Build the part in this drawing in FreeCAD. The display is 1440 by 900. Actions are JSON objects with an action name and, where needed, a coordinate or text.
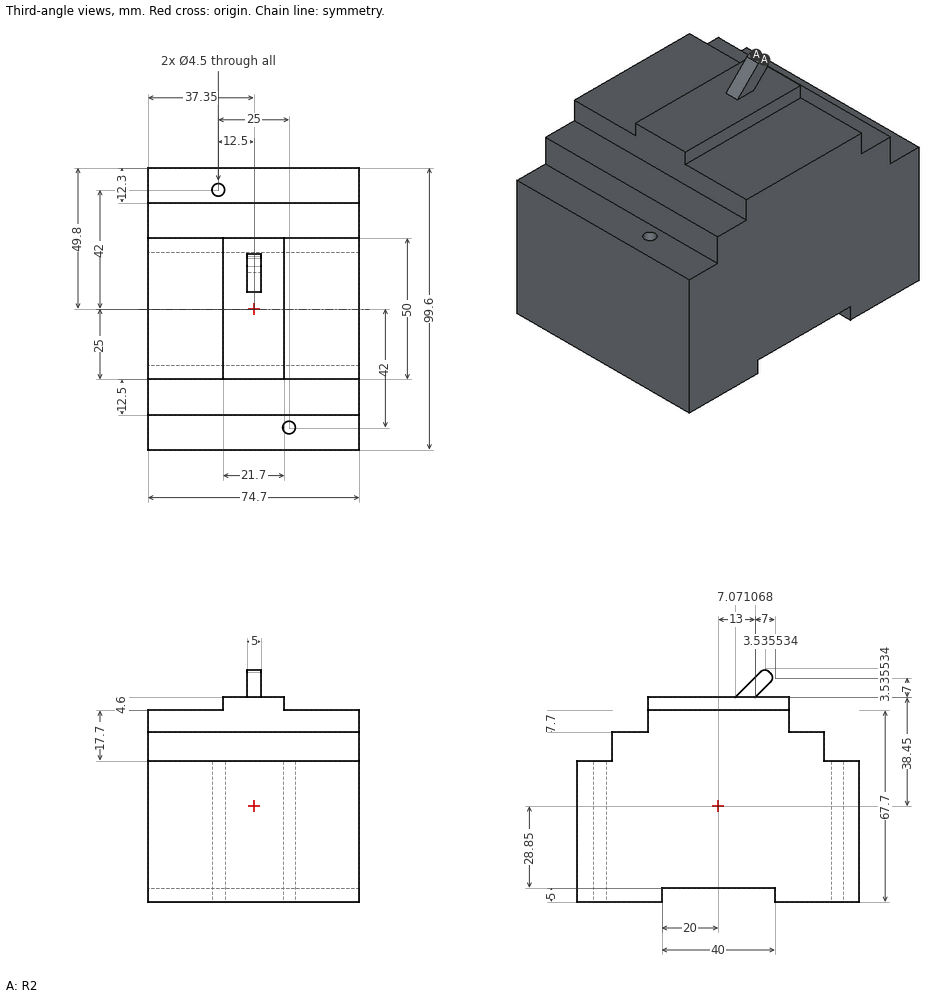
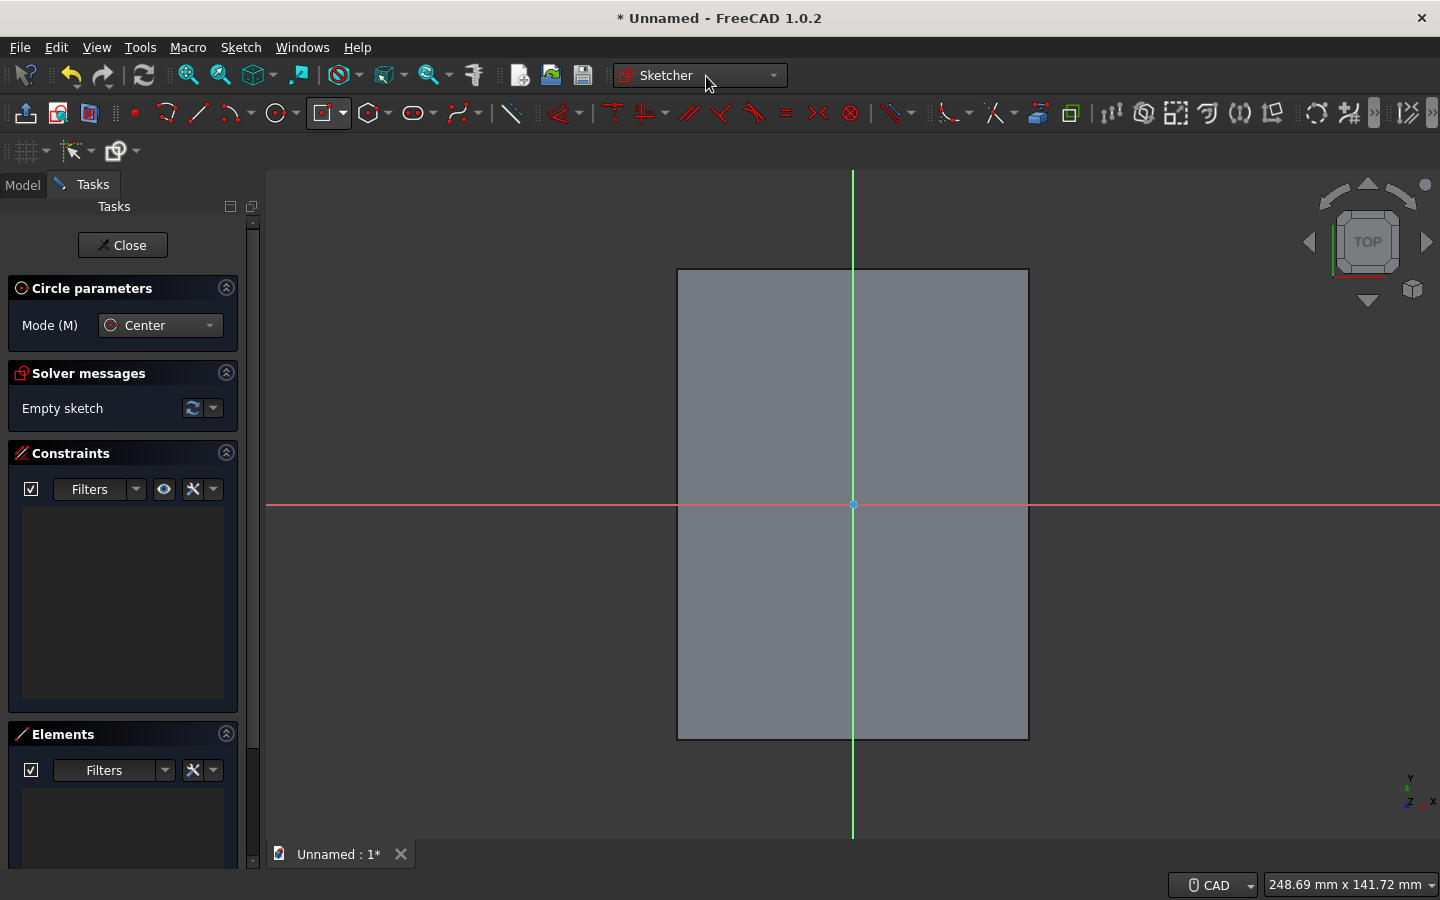
{"action": "scroll", "coordinate": [794, 306], "scroll_direction": "up", "scroll_amount": 4}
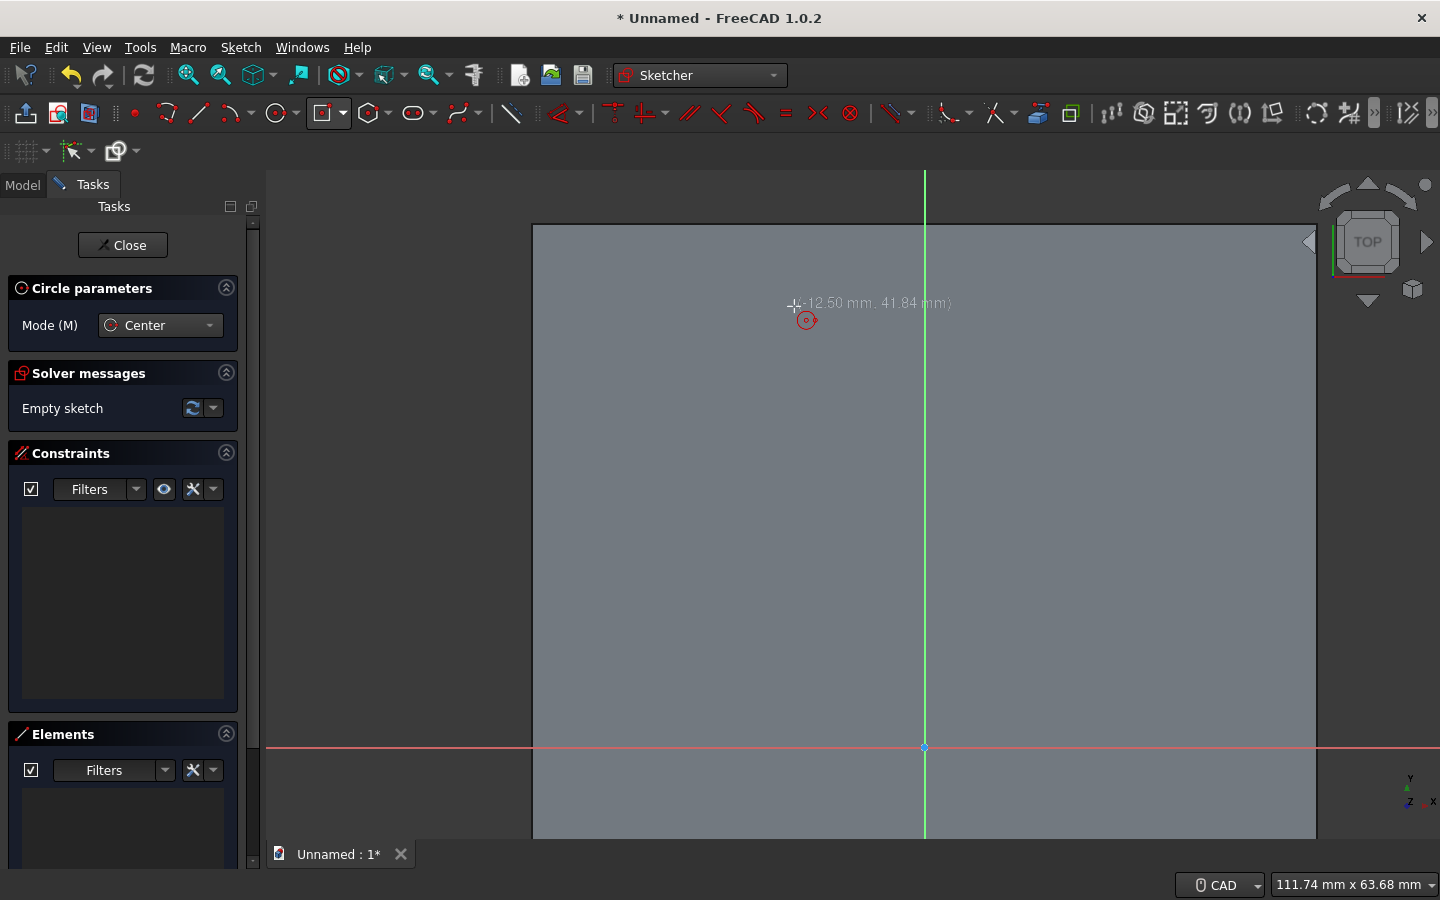
{"action": "left_click", "coordinate": [793, 306]}
{"action": "left_click", "coordinate": [810, 290]}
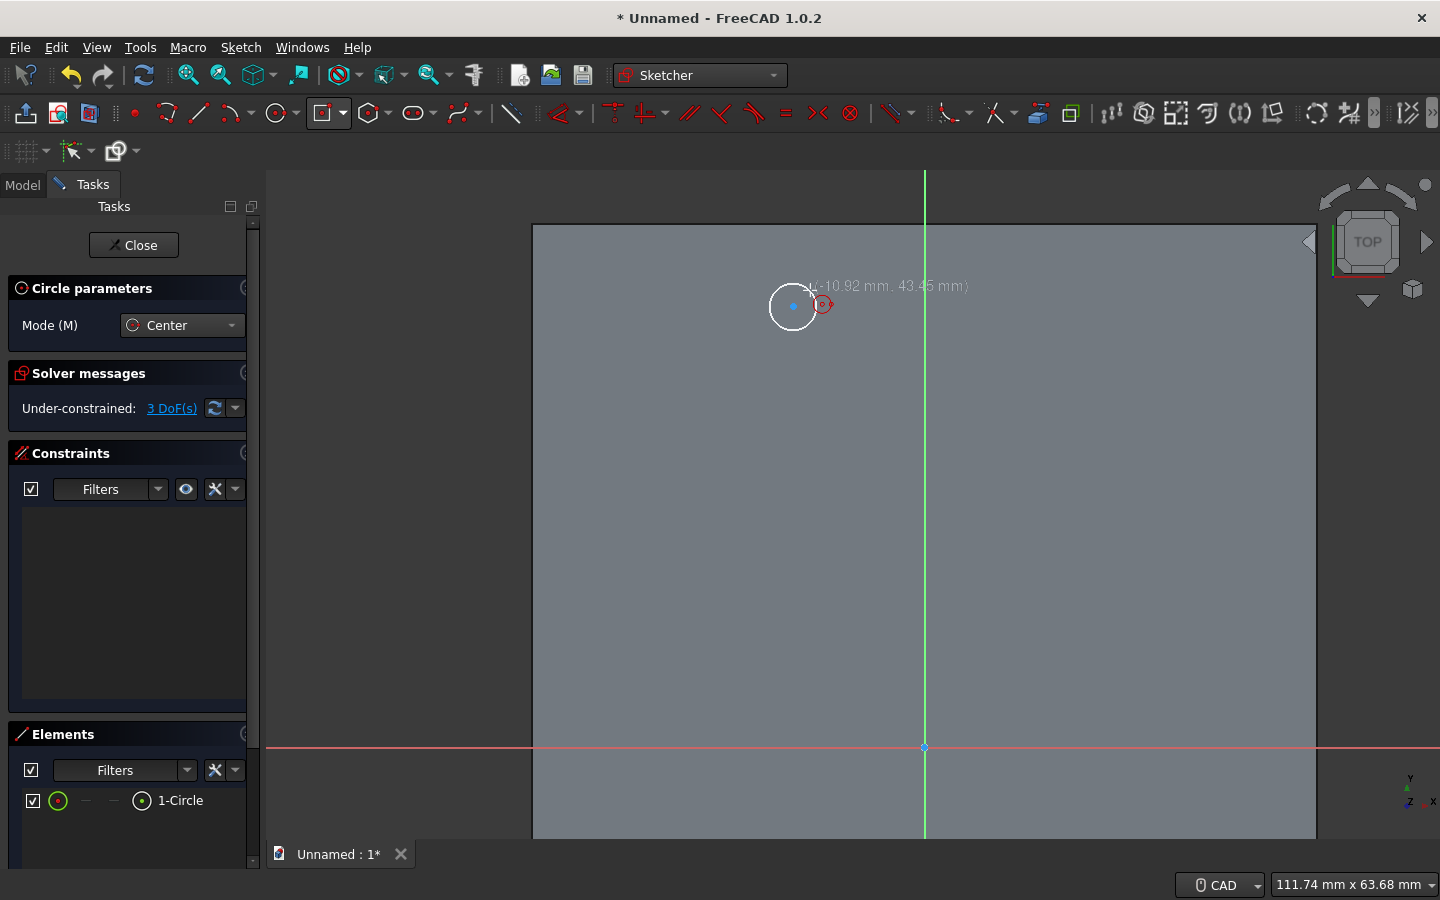
{"action": "scroll", "coordinate": [670, 306], "scroll_direction": "down", "scroll_amount": 4}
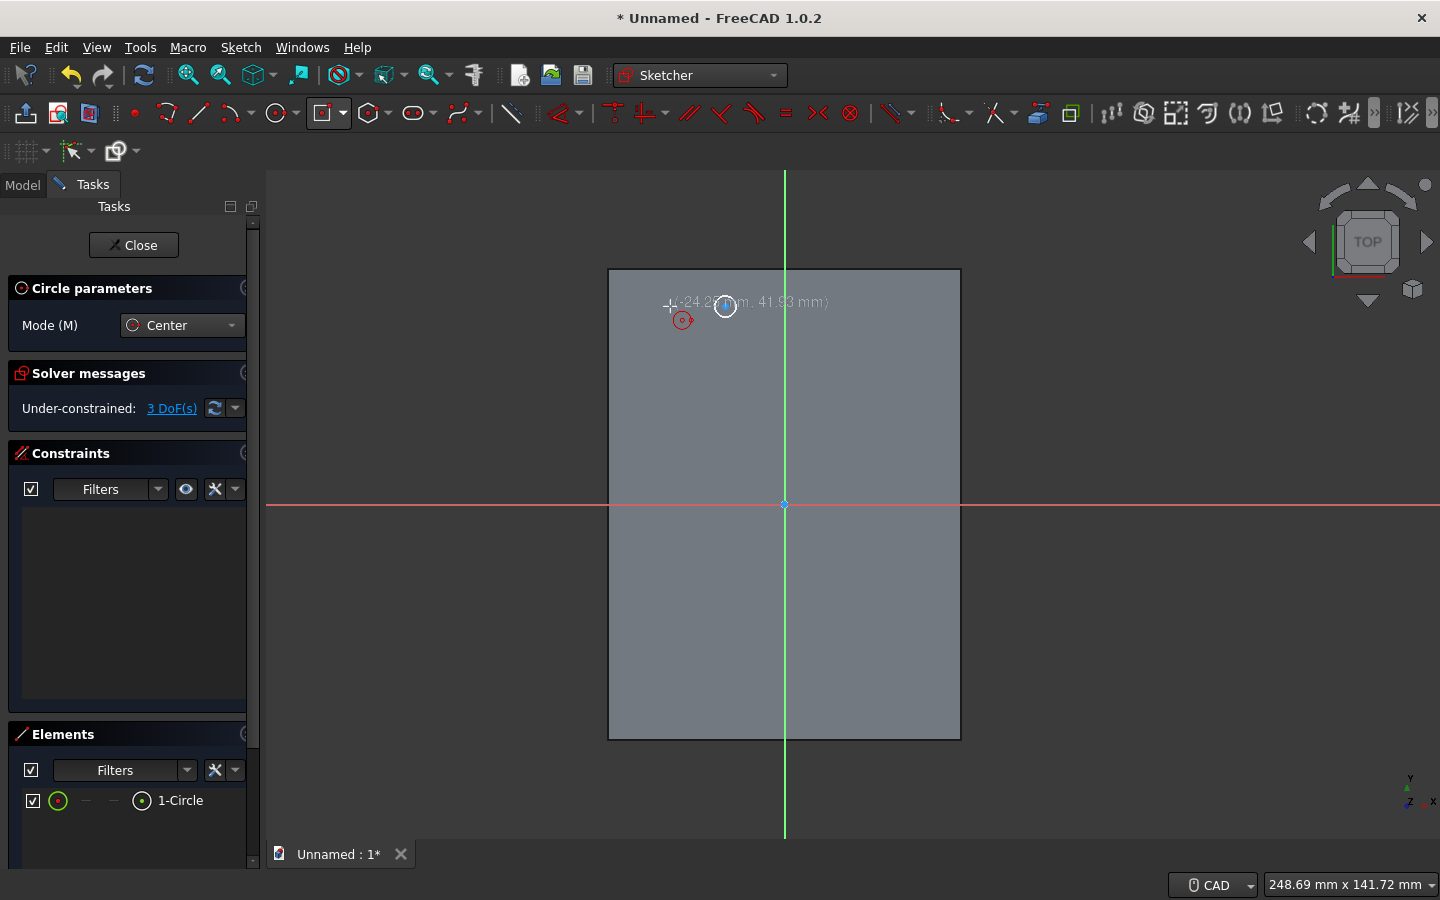
{"action": "scroll", "coordinate": [844, 703], "scroll_direction": "up", "scroll_amount": 4}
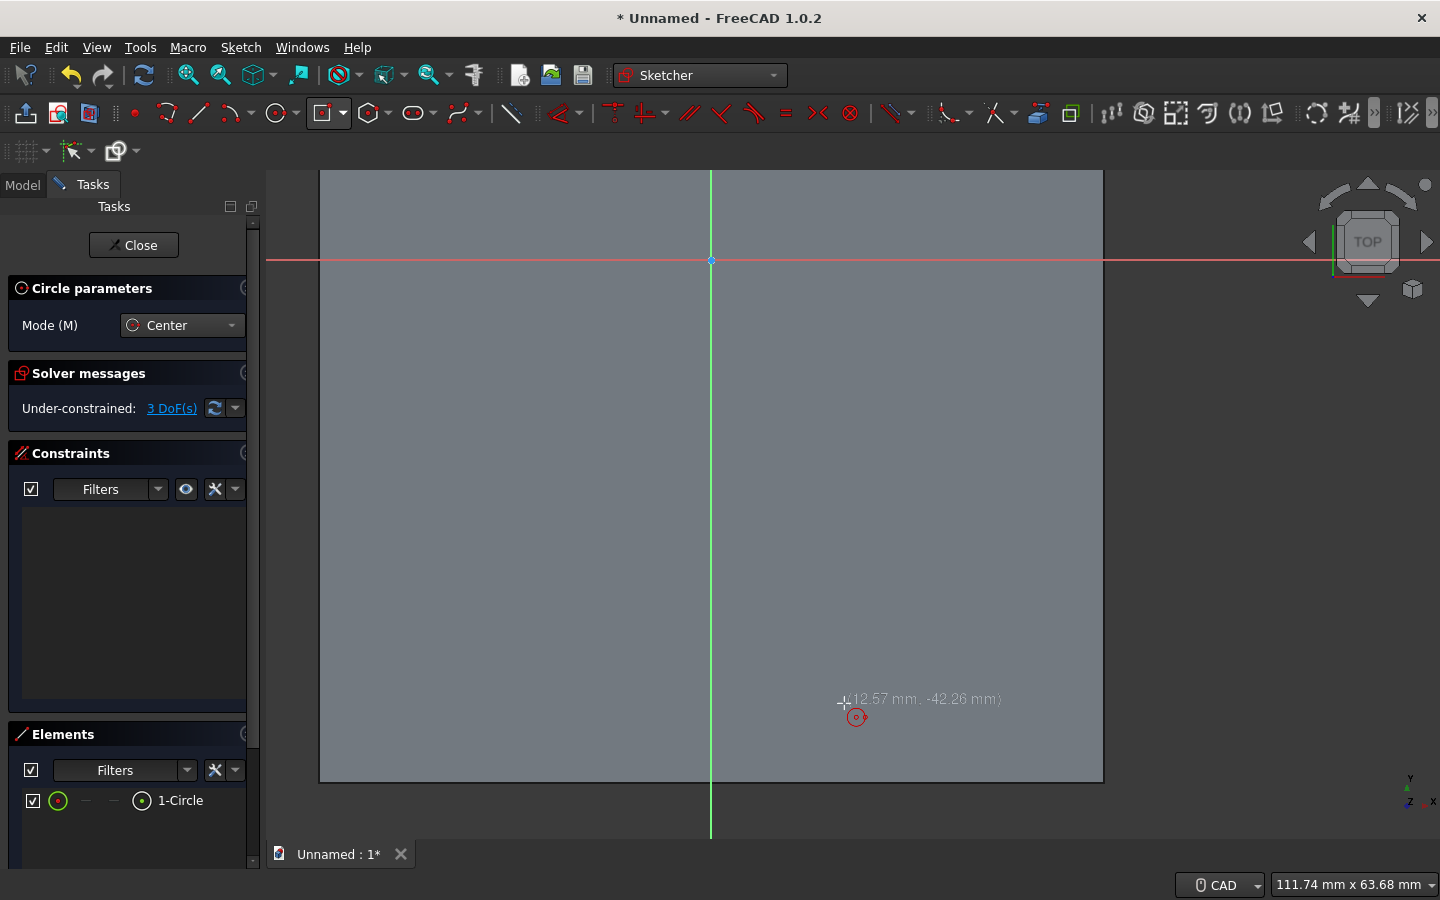
{"action": "left_click", "coordinate": [843, 702]}
{"action": "left_click", "coordinate": [859, 685]}
{"action": "key", "text": "Escape"}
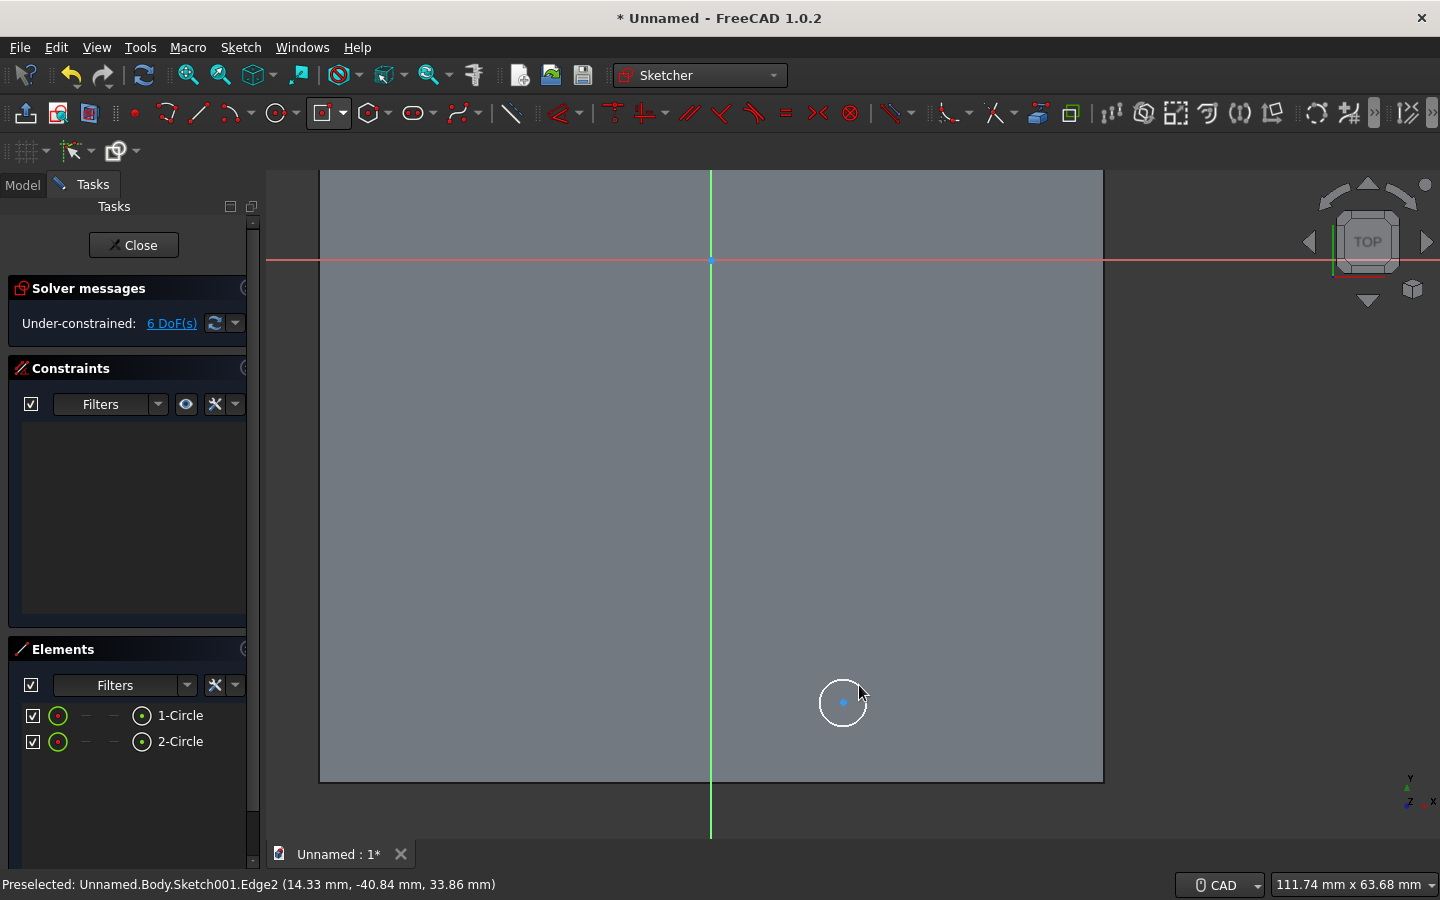
{"action": "scroll", "coordinate": [844, 704], "scroll_direction": "down", "scroll_amount": 4}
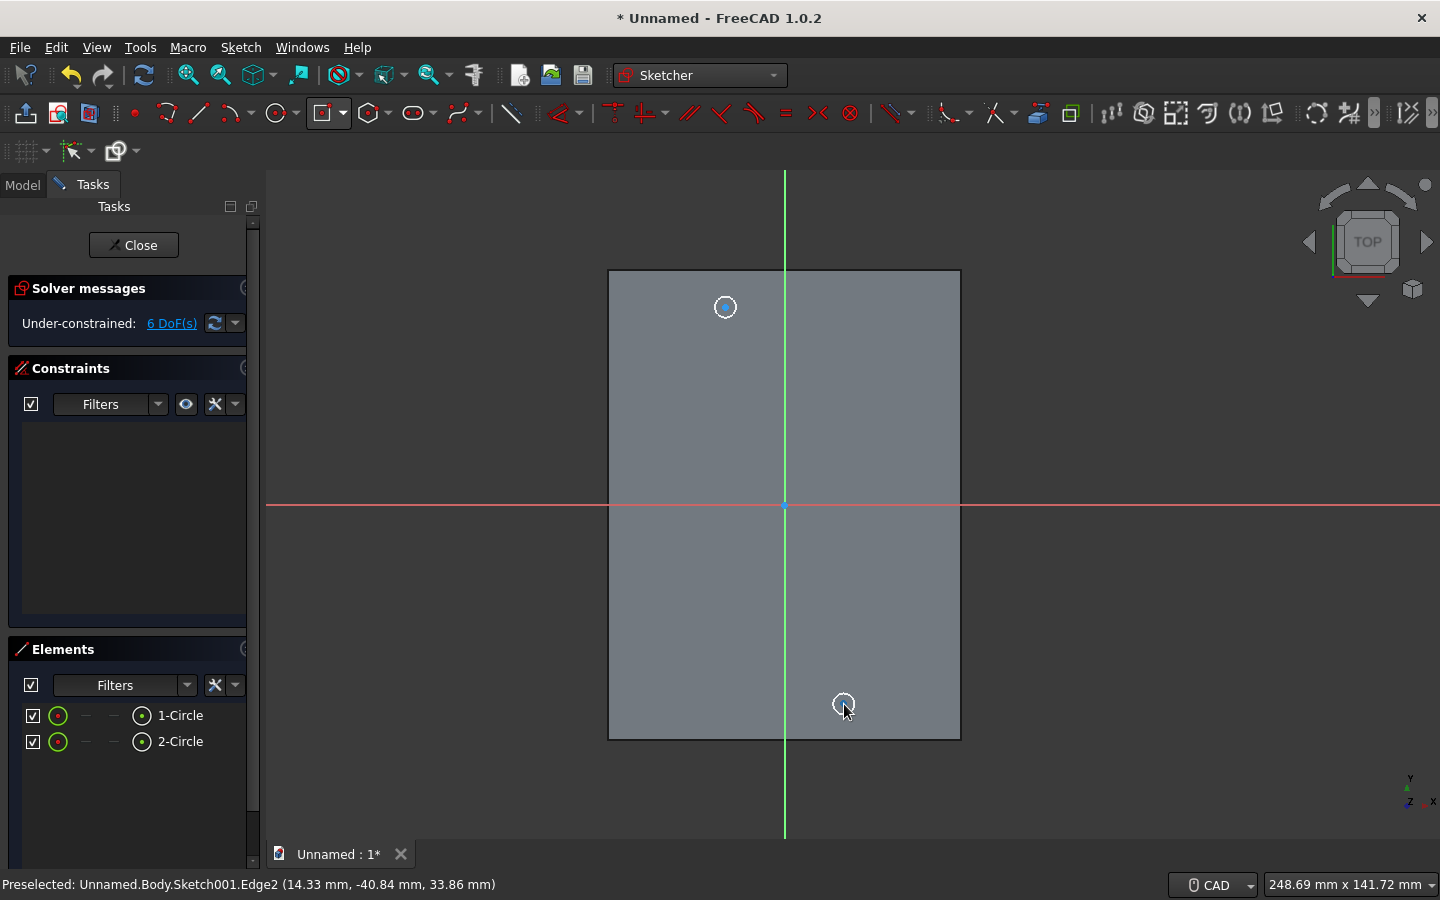
{"action": "scroll", "coordinate": [733, 300], "scroll_direction": "up", "scroll_amount": 2}